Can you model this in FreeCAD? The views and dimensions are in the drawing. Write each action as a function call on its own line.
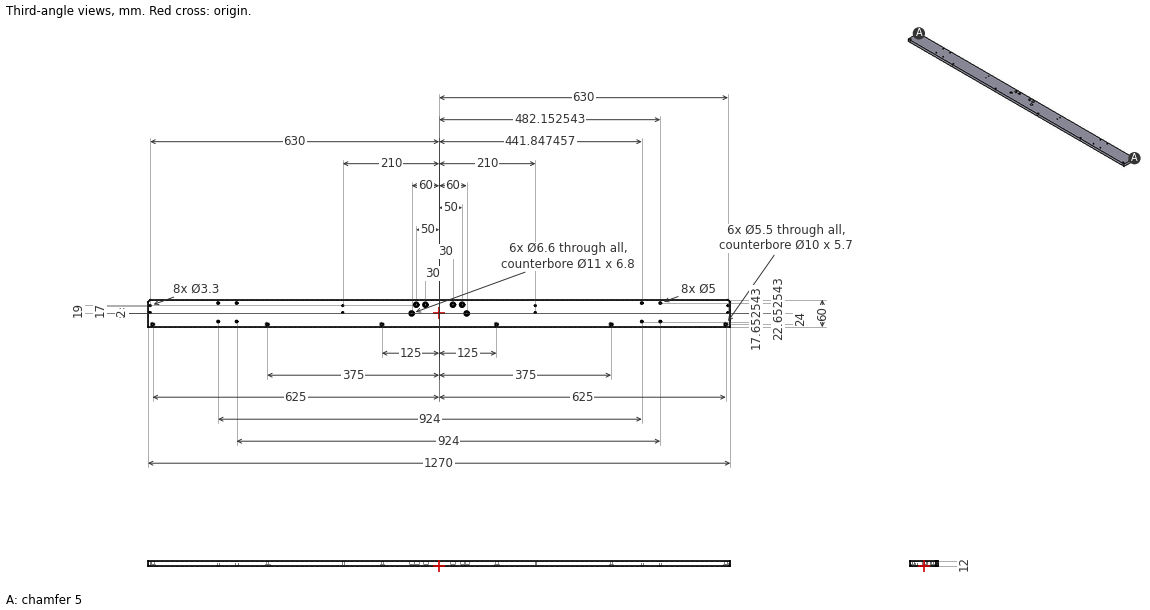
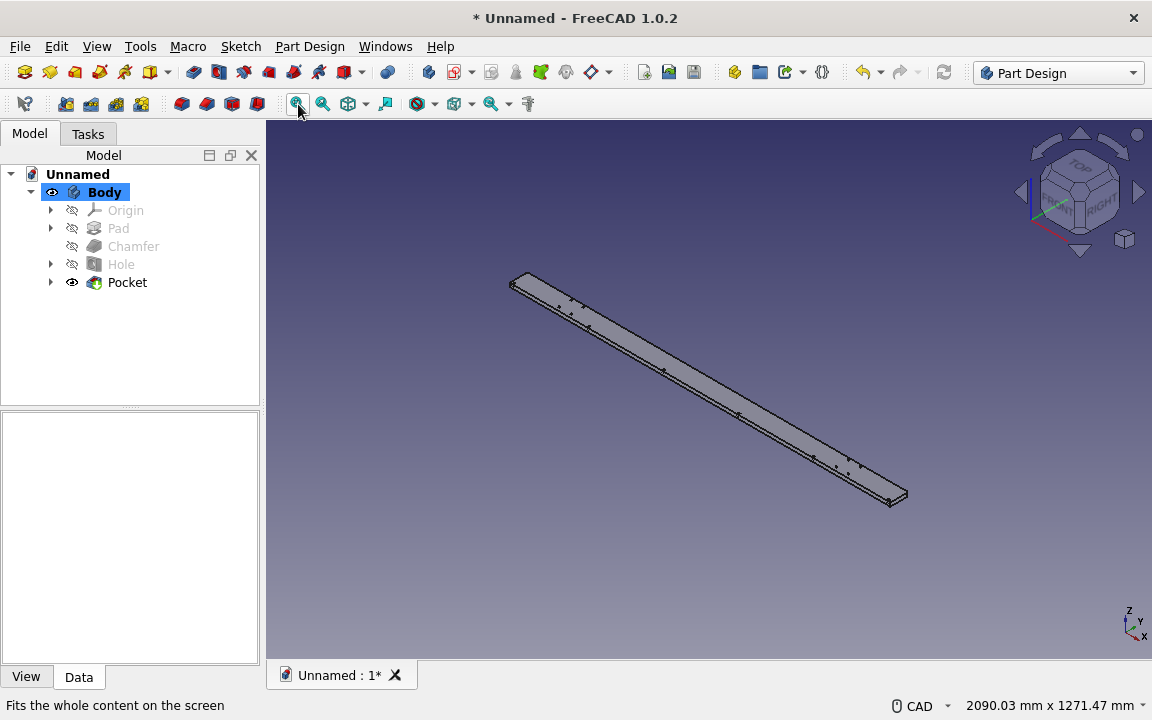
click(709, 386)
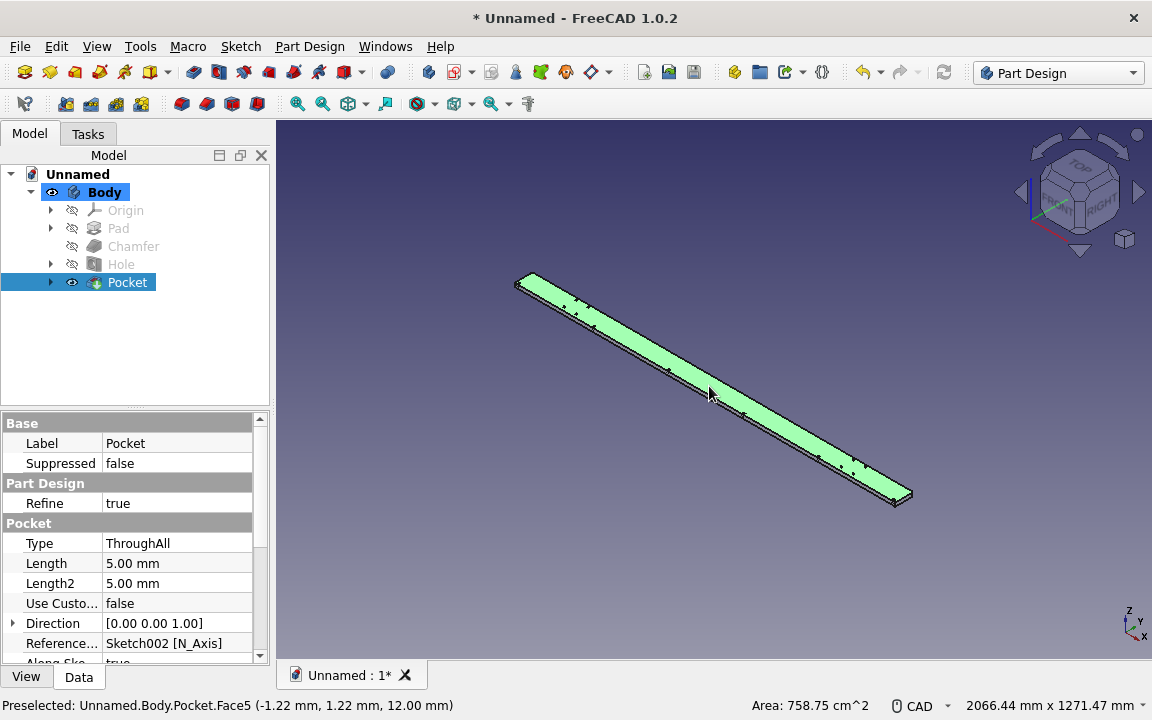
click(454, 72)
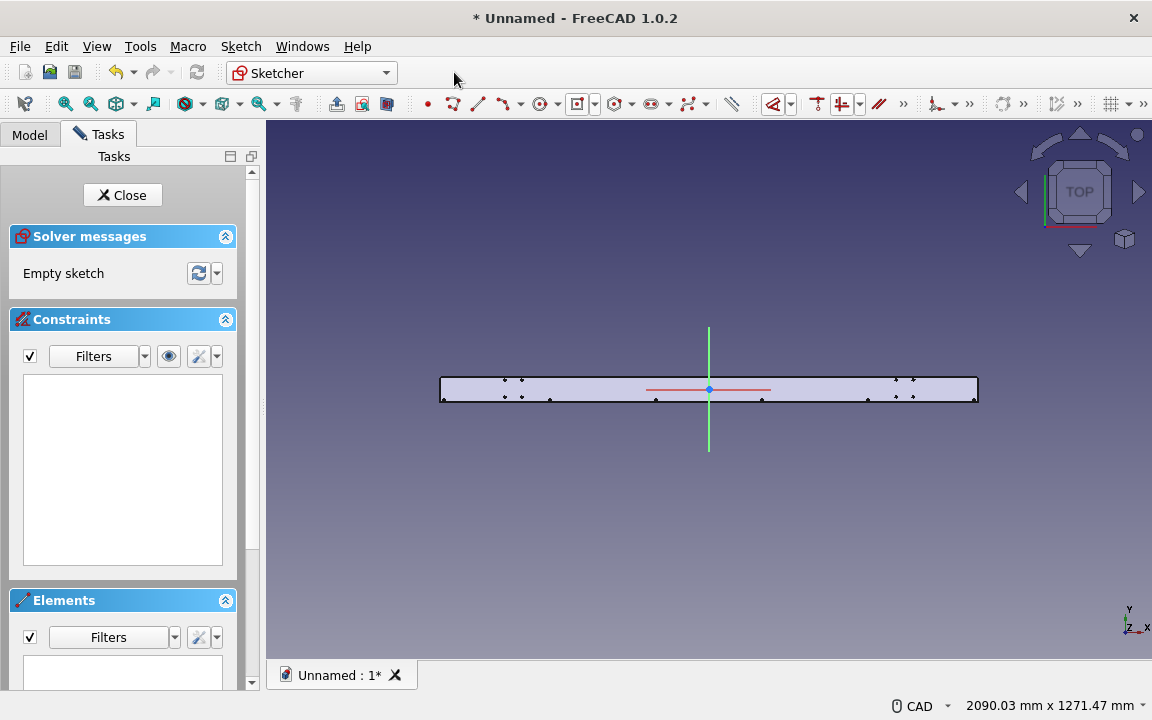
scroll(331, 407, down, 1)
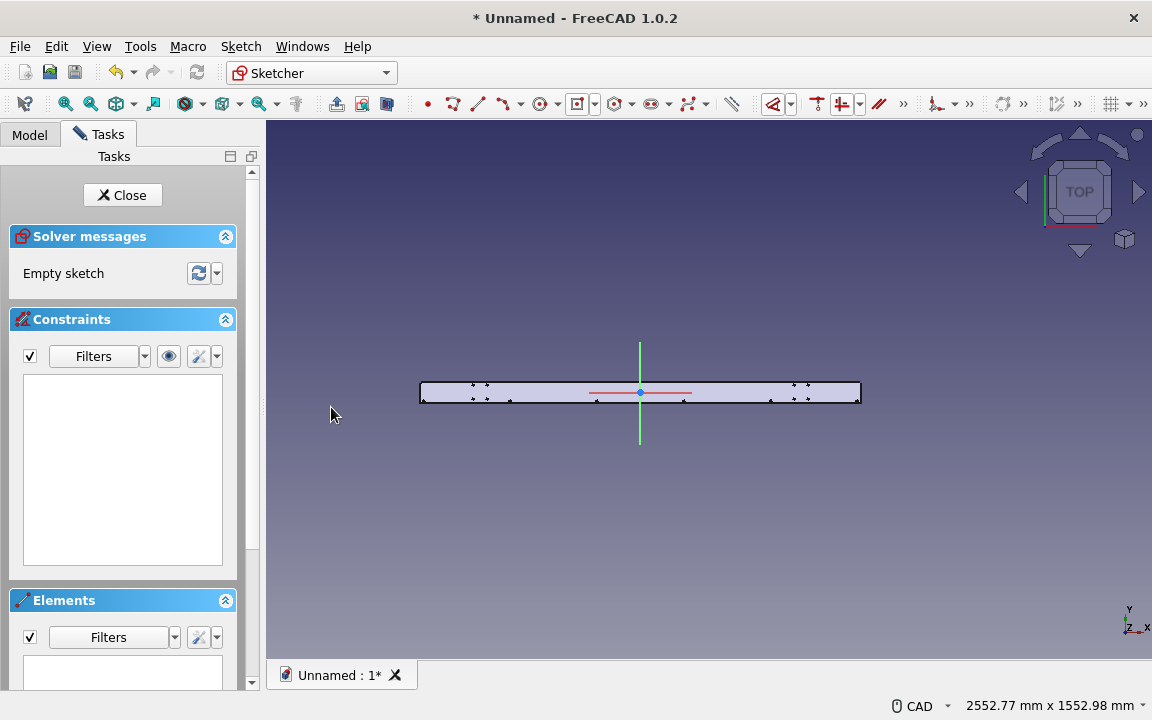
click(540, 104)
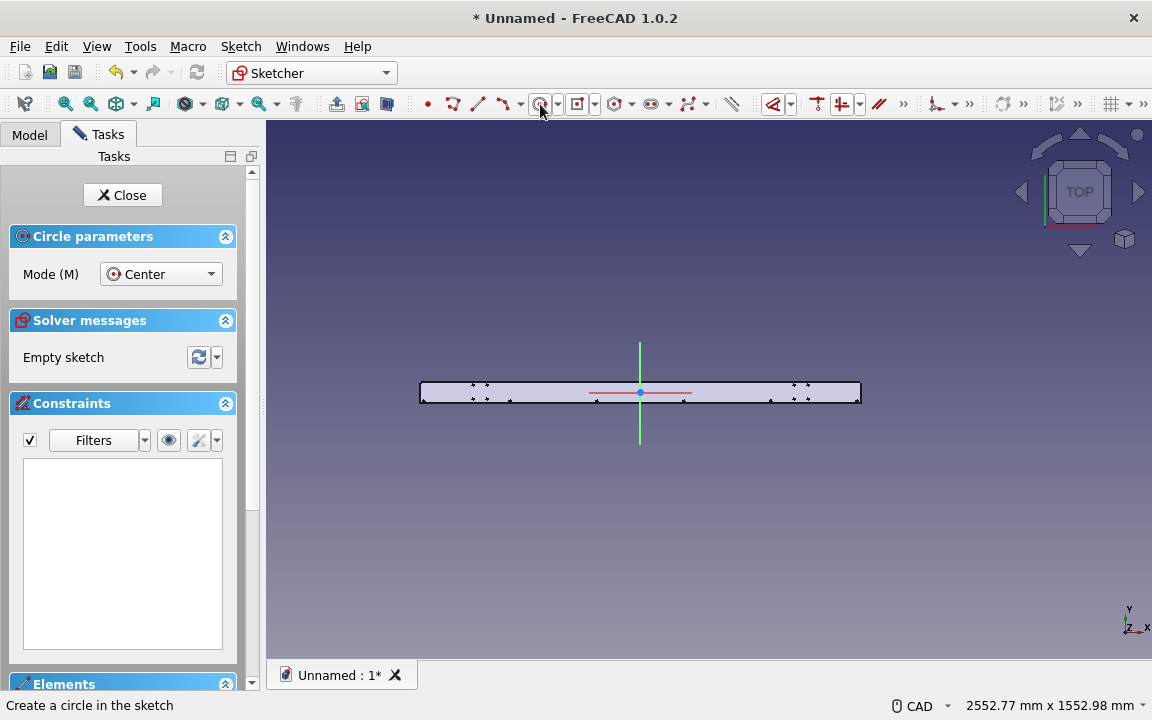
scroll(422, 387, up, 19)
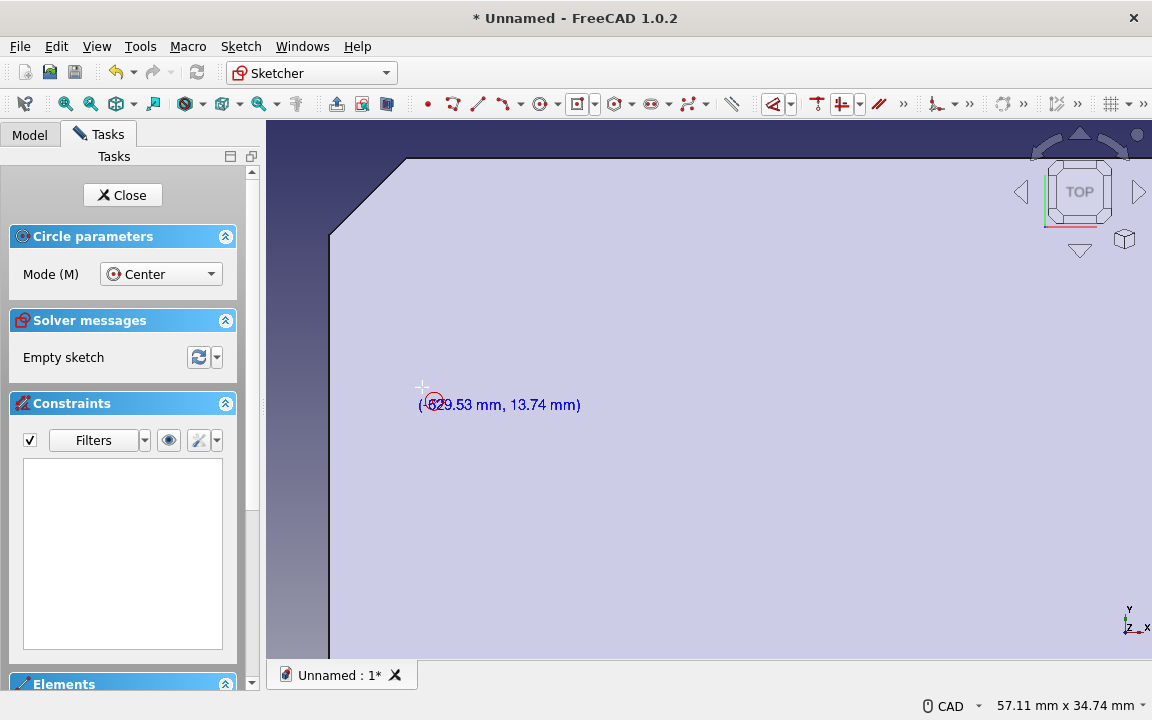
scroll(372, 387, down, 18)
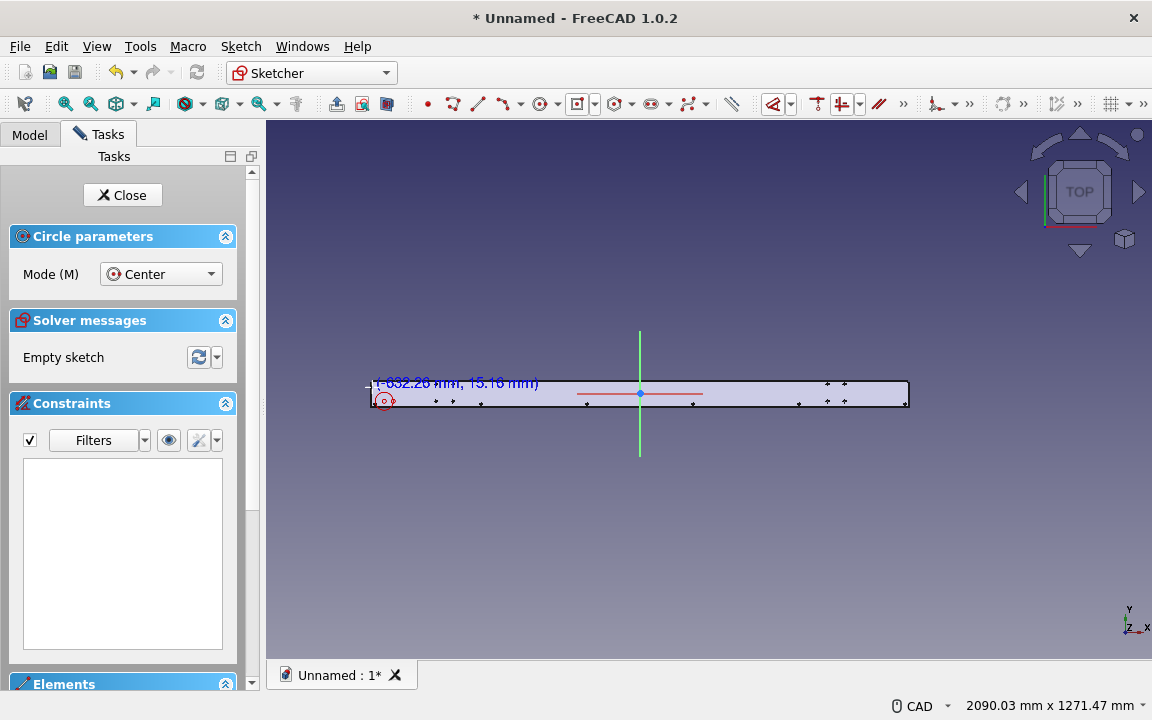
scroll(373, 387, up, 4)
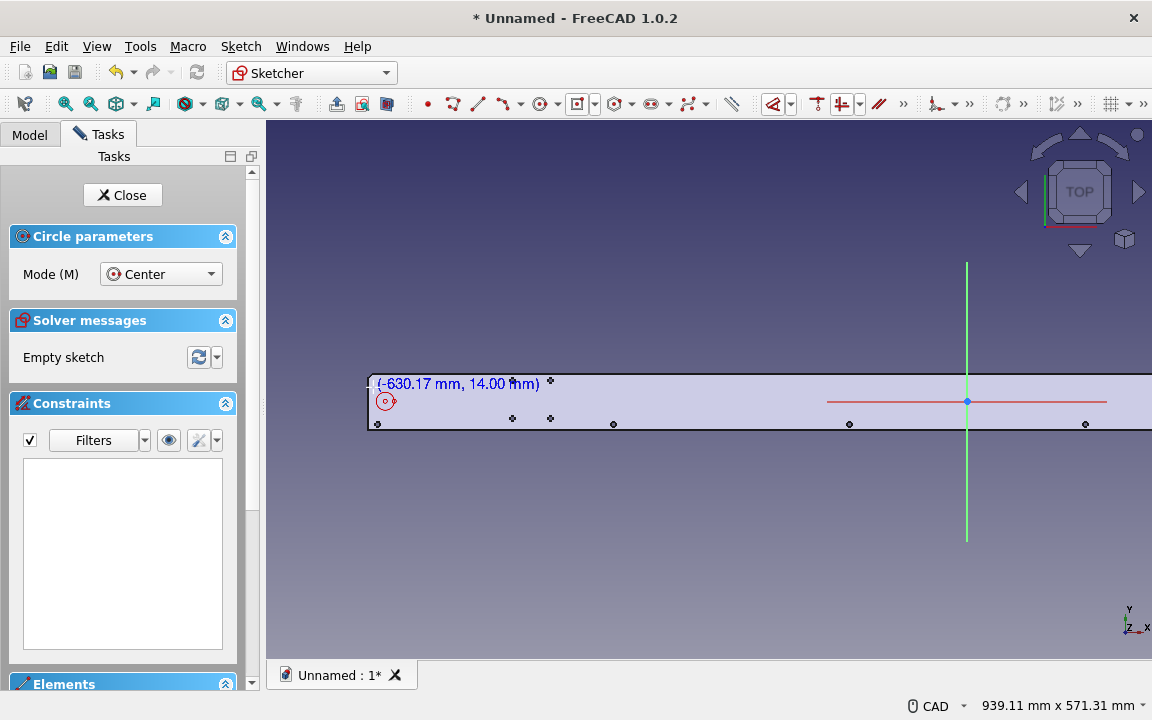
click(373, 386)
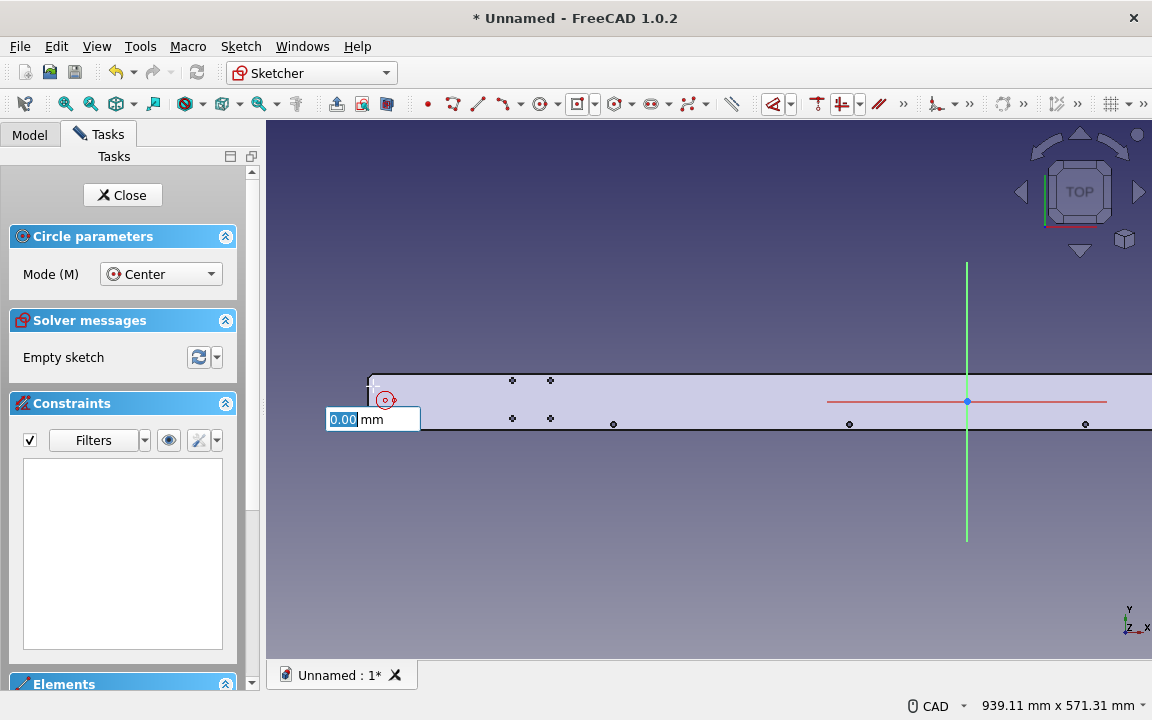
scroll(374, 385, up, 12)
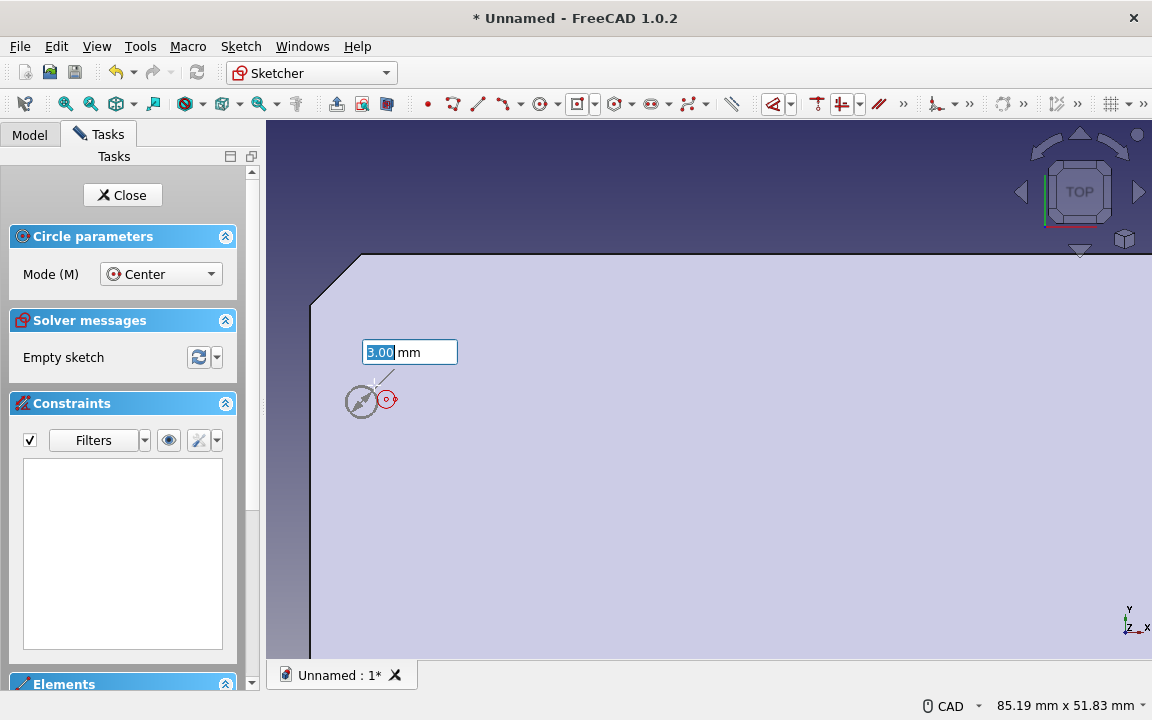
click(374, 377)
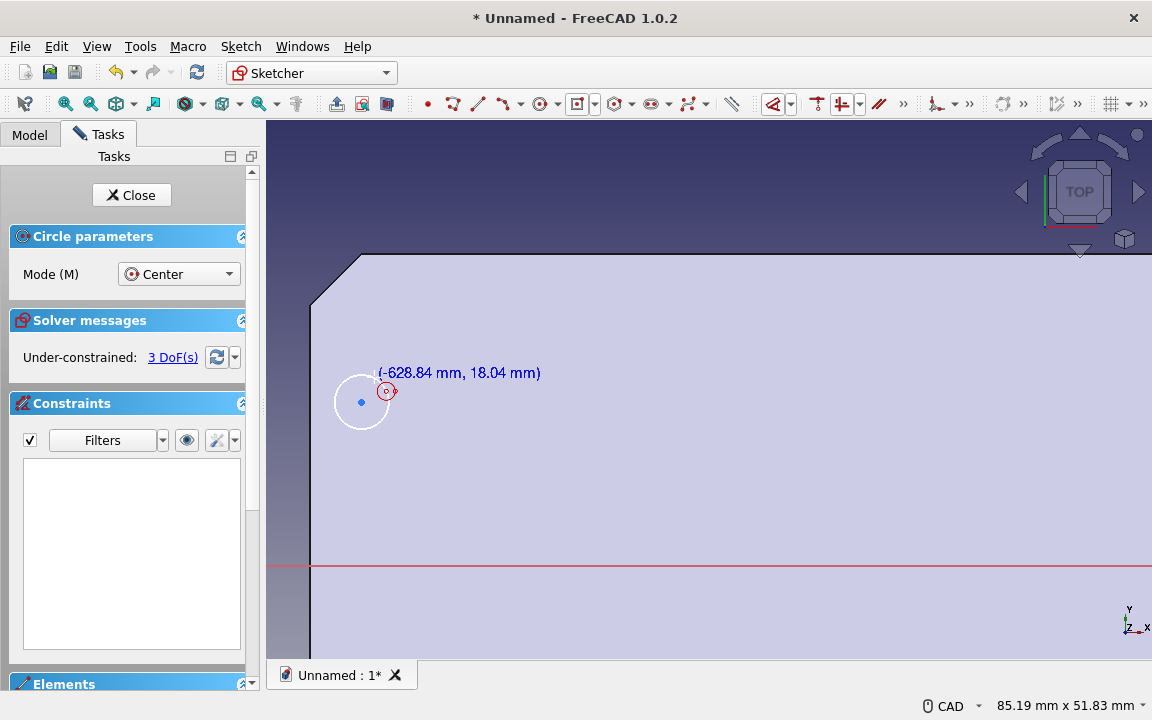
scroll(362, 545, up, 2)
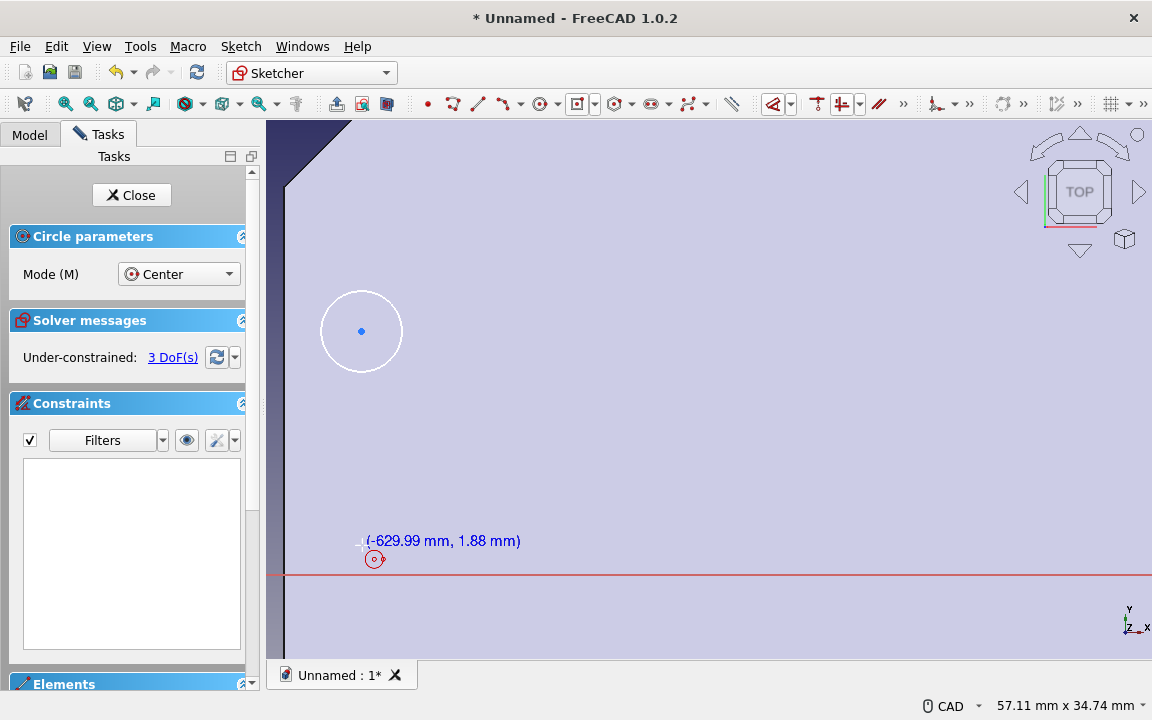
click(362, 544)
click(380, 526)